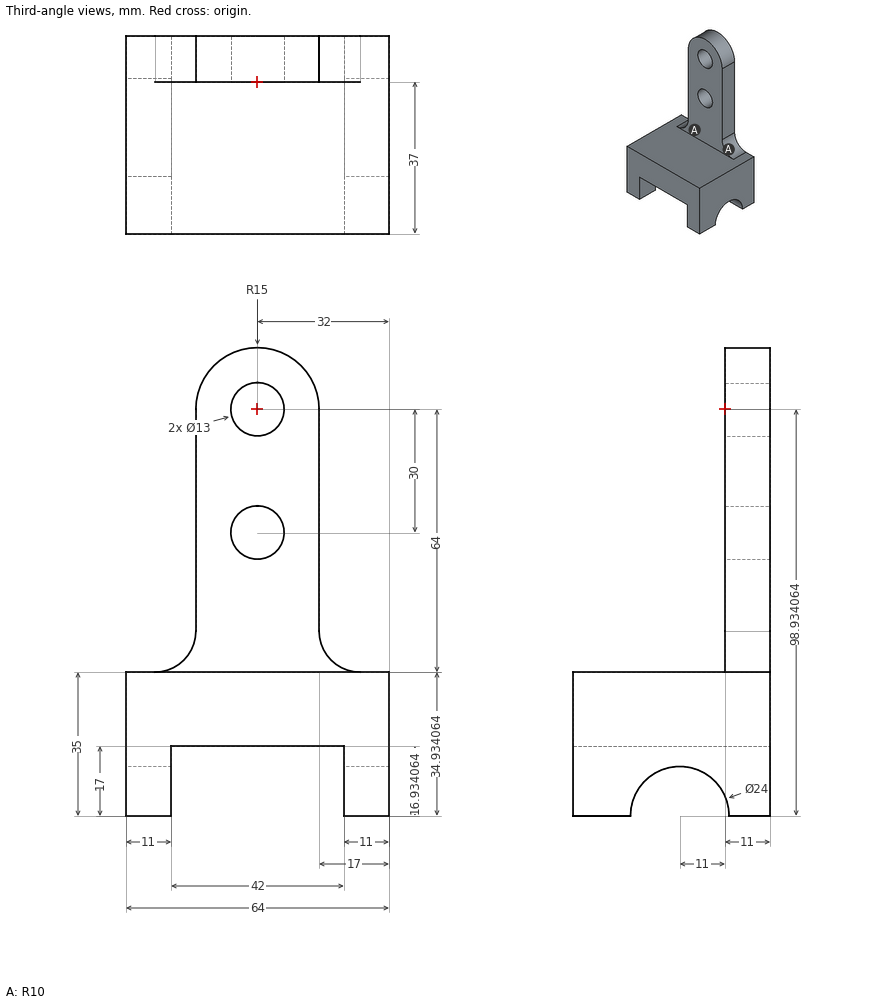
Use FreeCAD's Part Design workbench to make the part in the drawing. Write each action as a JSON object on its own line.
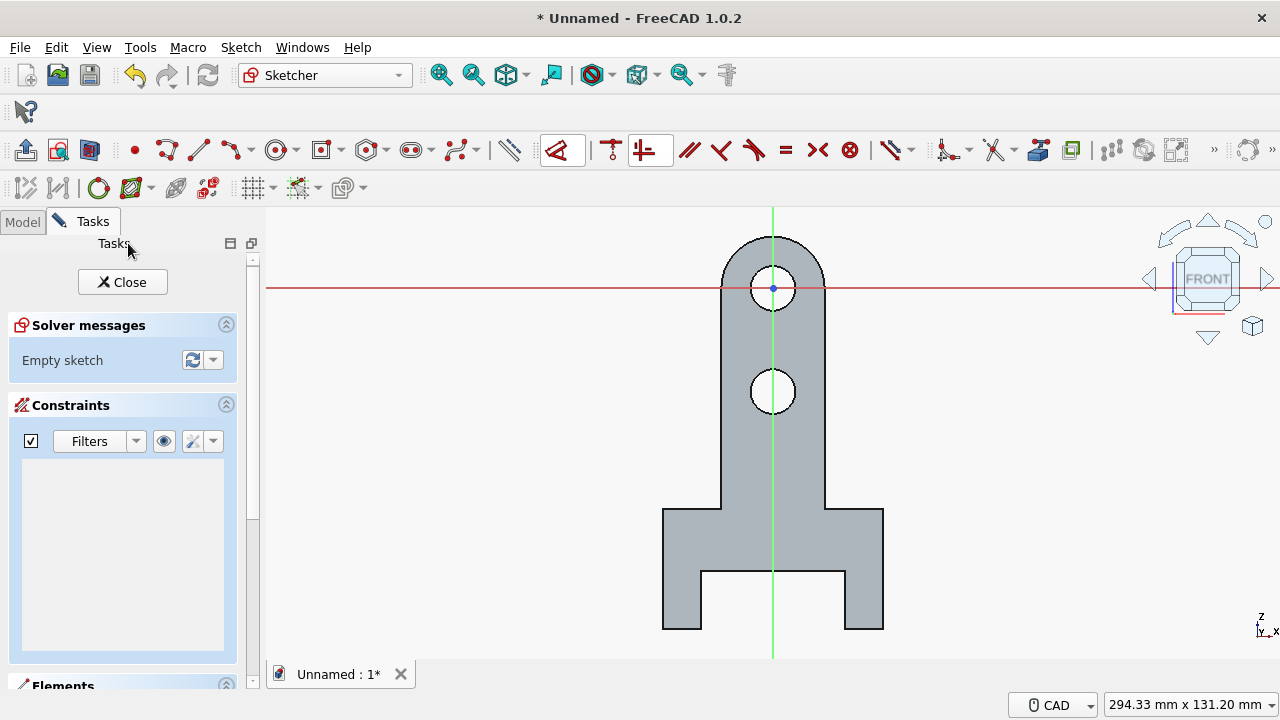
{"action": "scroll", "coordinate": [395, 316], "scroll_direction": "down", "scroll_amount": 1}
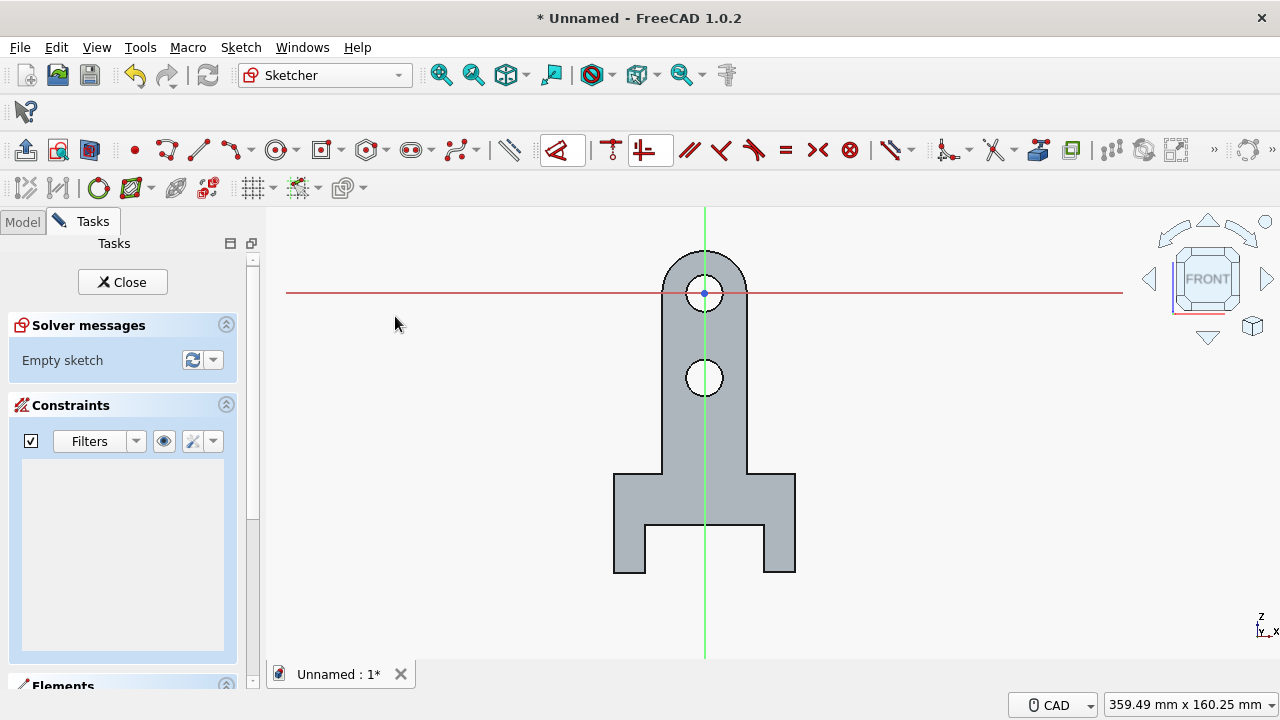
{"action": "left_click", "coordinate": [168, 150]}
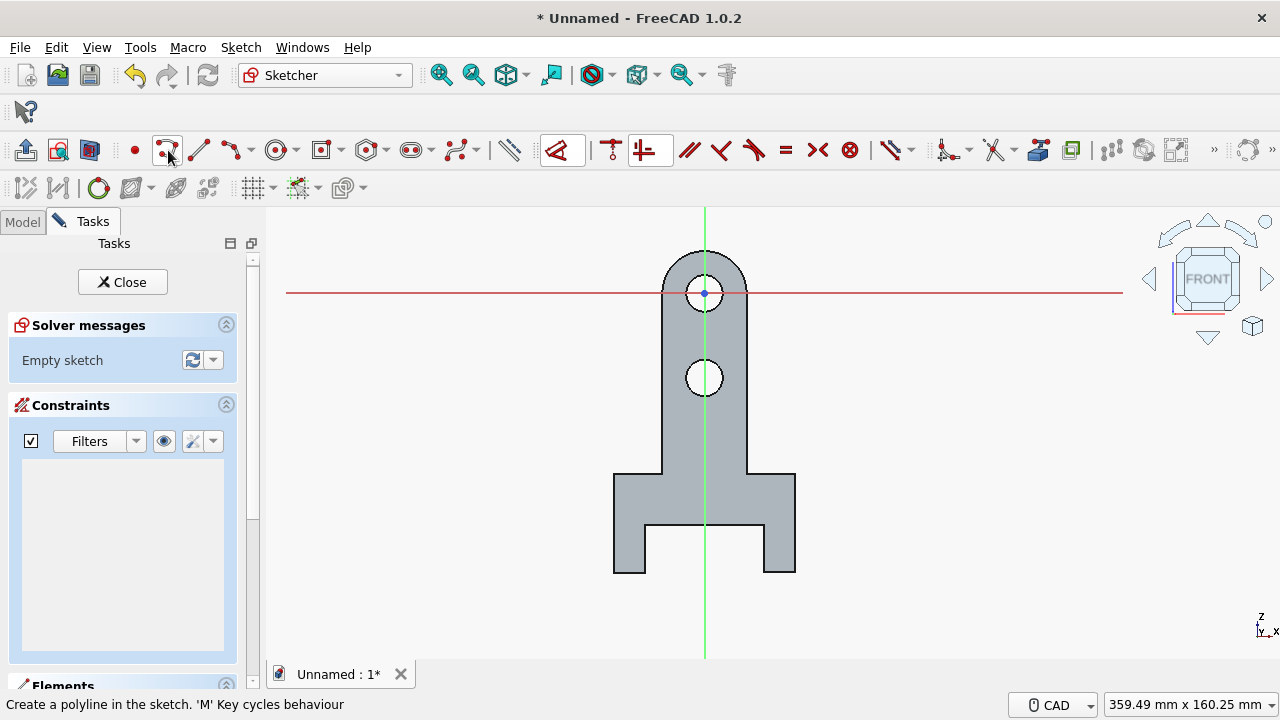
{"action": "left_click", "coordinate": [795, 474]}
{"action": "left_click", "coordinate": [614, 474]}
{"action": "left_click", "coordinate": [614, 573]}
{"action": "left_click", "coordinate": [645, 573]}
{"action": "left_click", "coordinate": [645, 525]}
{"action": "left_click", "coordinate": [764, 525]}
{"action": "left_click", "coordinate": [764, 572]}
{"action": "left_click", "coordinate": [795, 572]}
{"action": "left_click", "coordinate": [795, 475]}
{"action": "key", "text": "Escape"}
{"action": "key", "text": "Escape"}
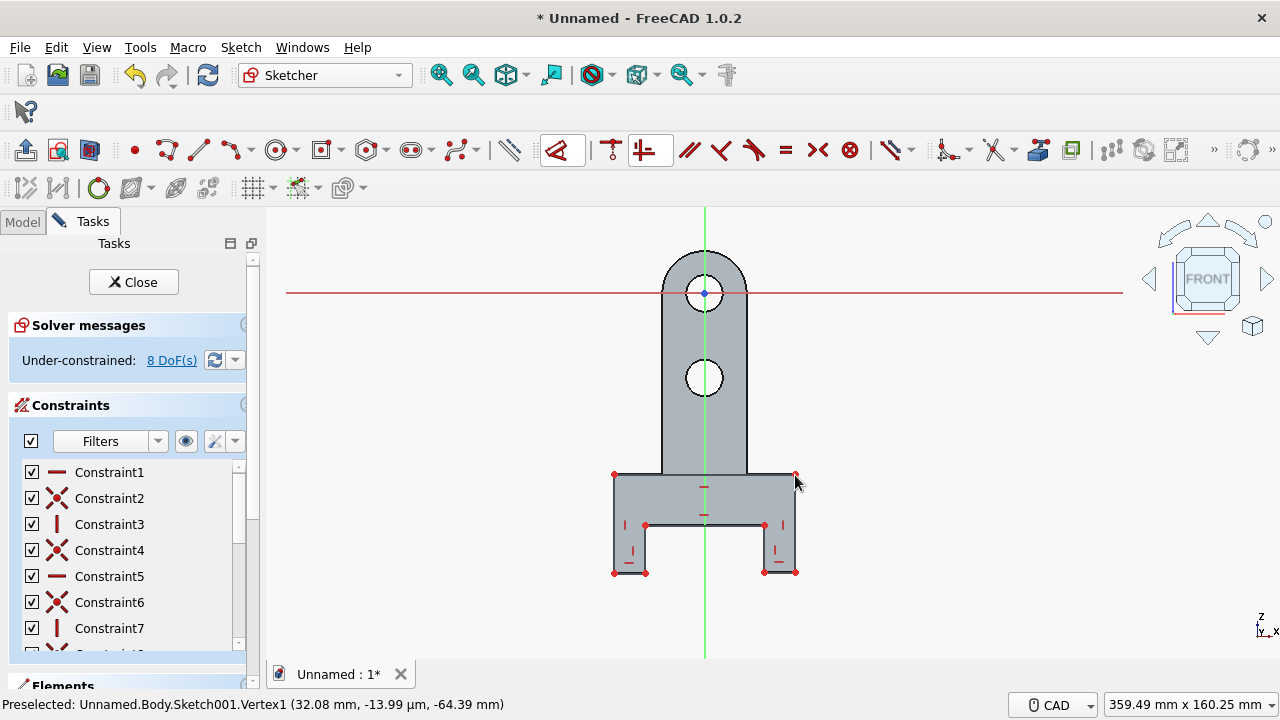
{"action": "left_click", "coordinate": [741, 475]}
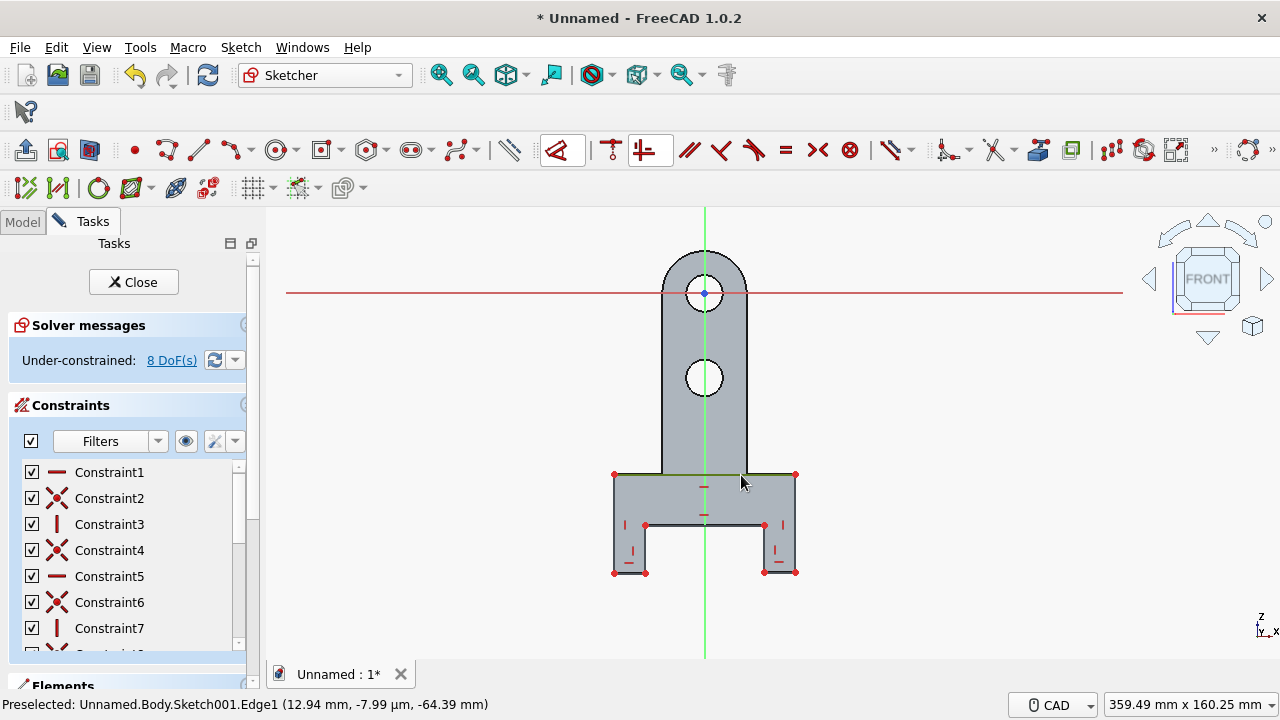
{"action": "key", "text": "l"}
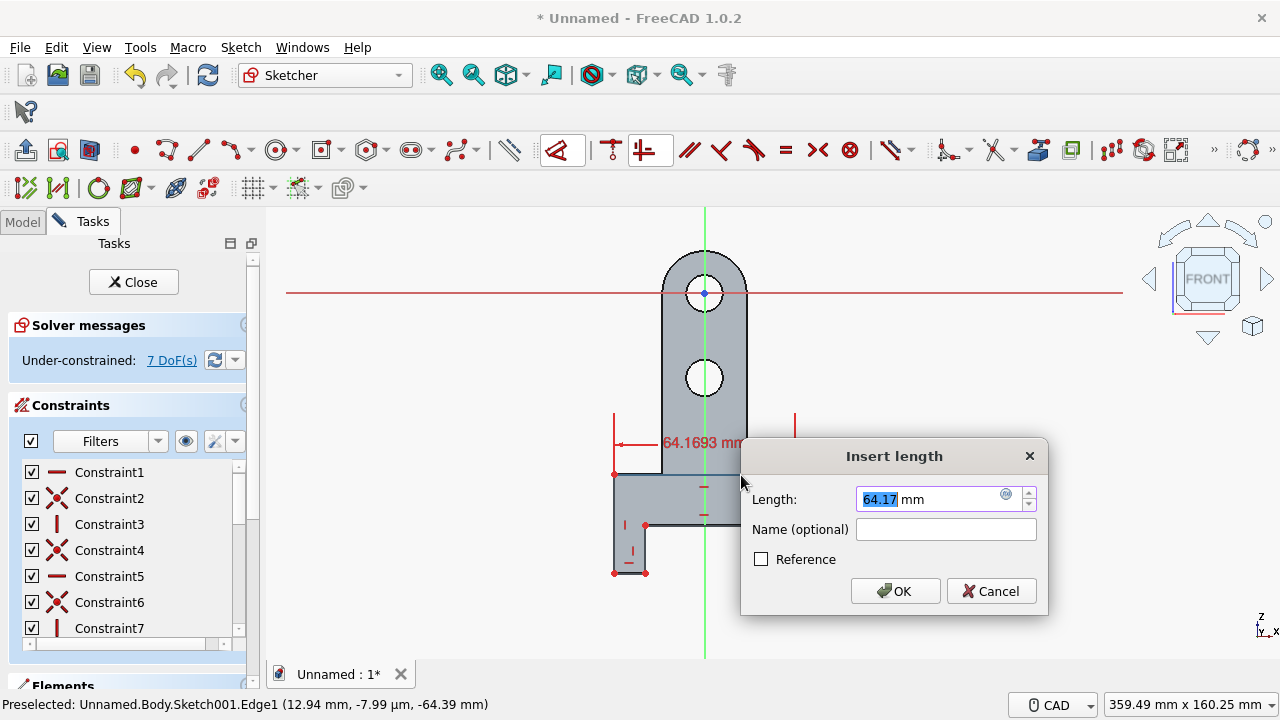
{"action": "type", "text": "64"}
{"action": "key", "text": "Return"}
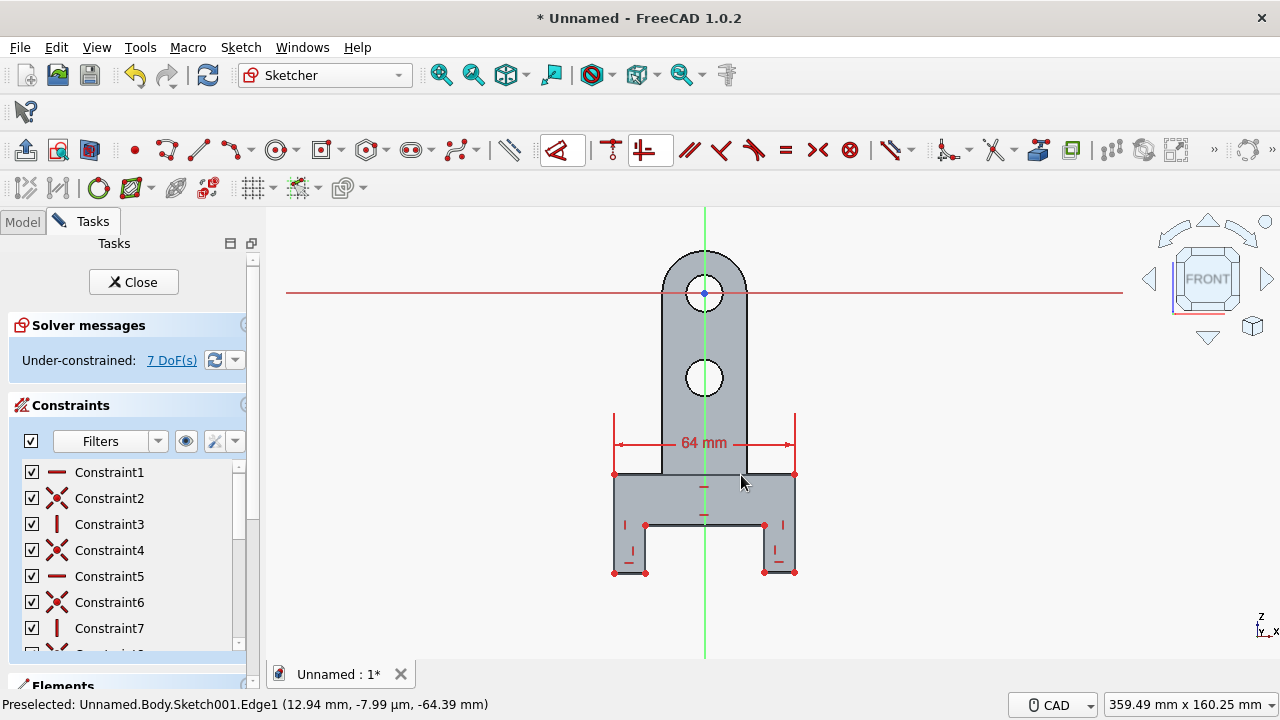
{"action": "left_click", "coordinate": [614, 505]}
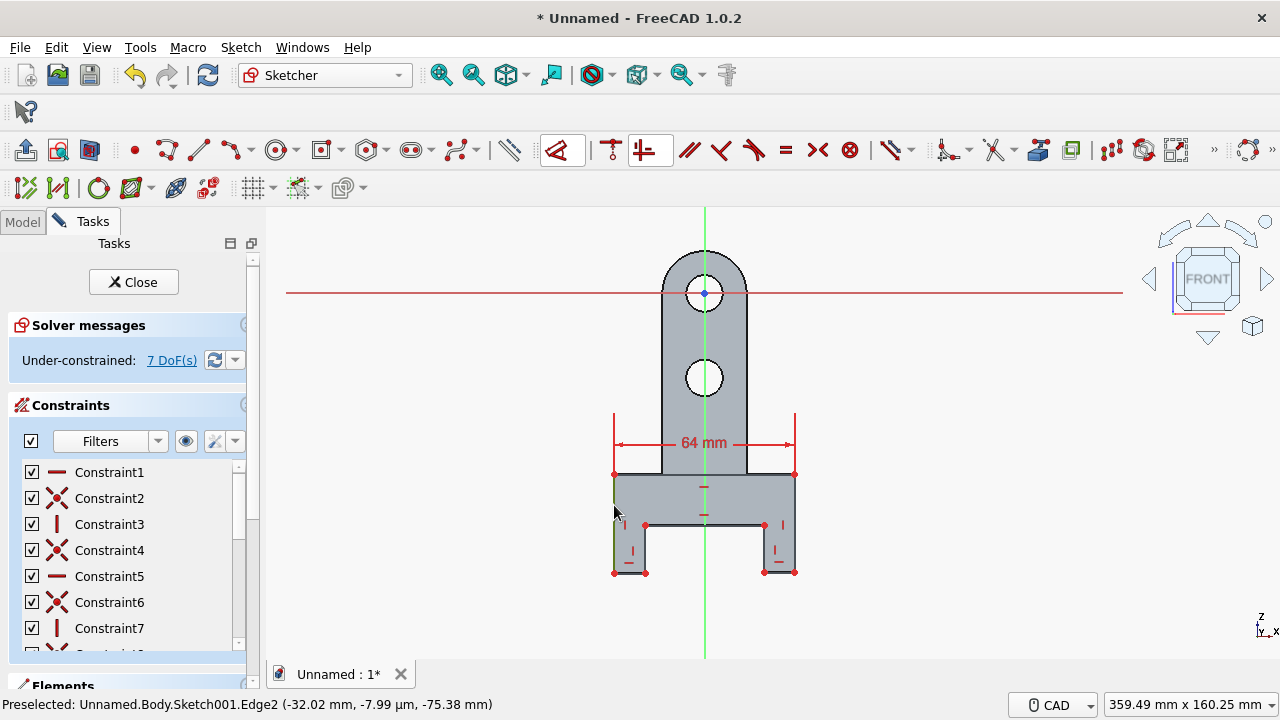
{"action": "left_click", "coordinate": [580, 150]}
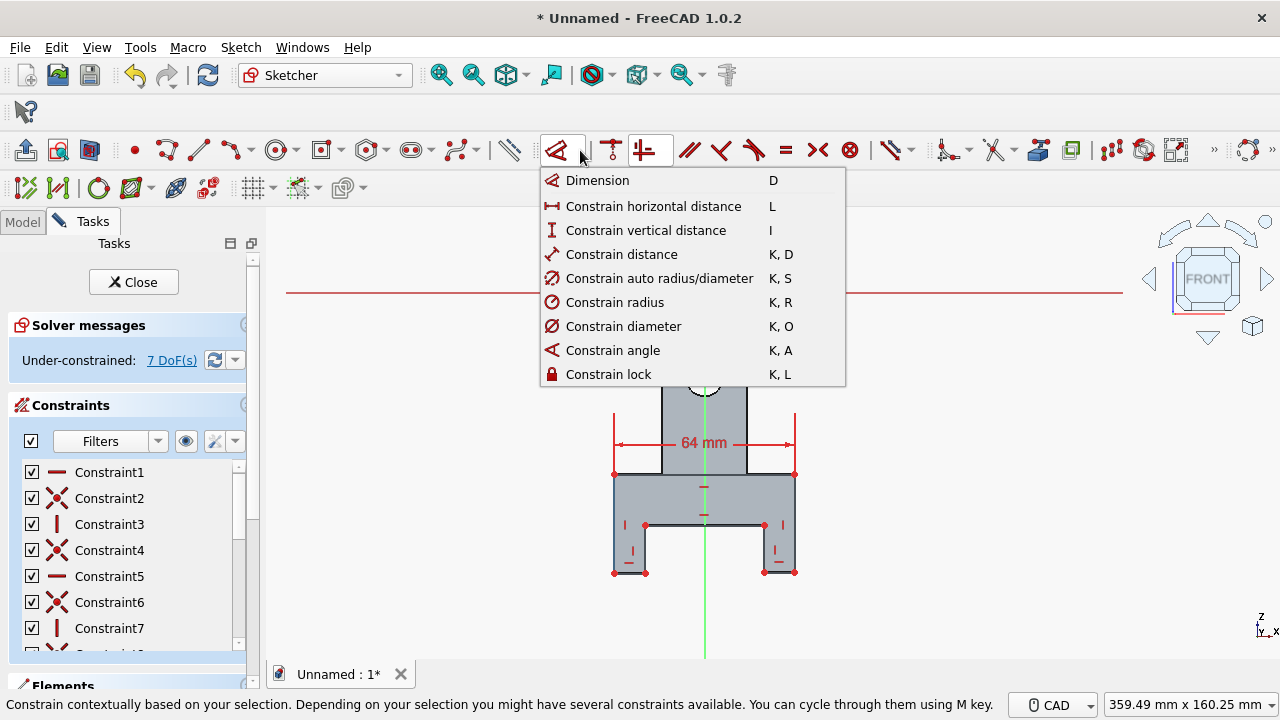
{"action": "left_click", "coordinate": [693, 230]}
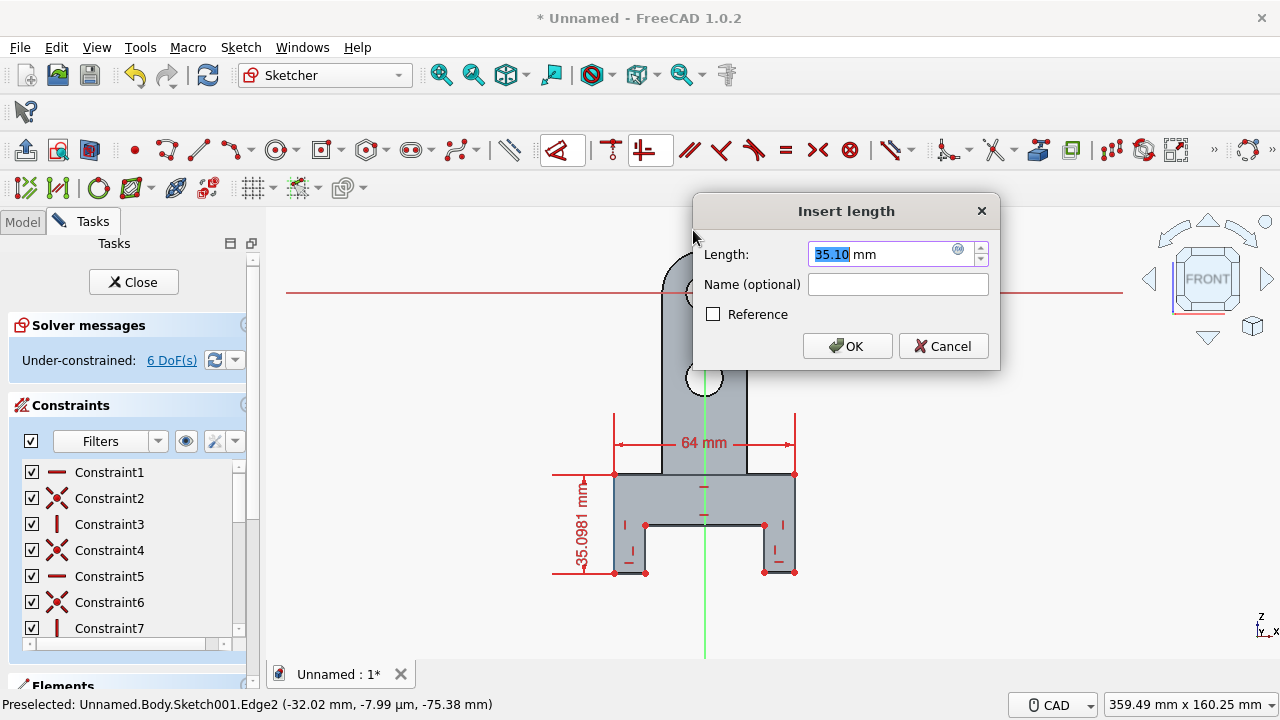
{"action": "type", "text": "35"}
{"action": "key", "text": "Return"}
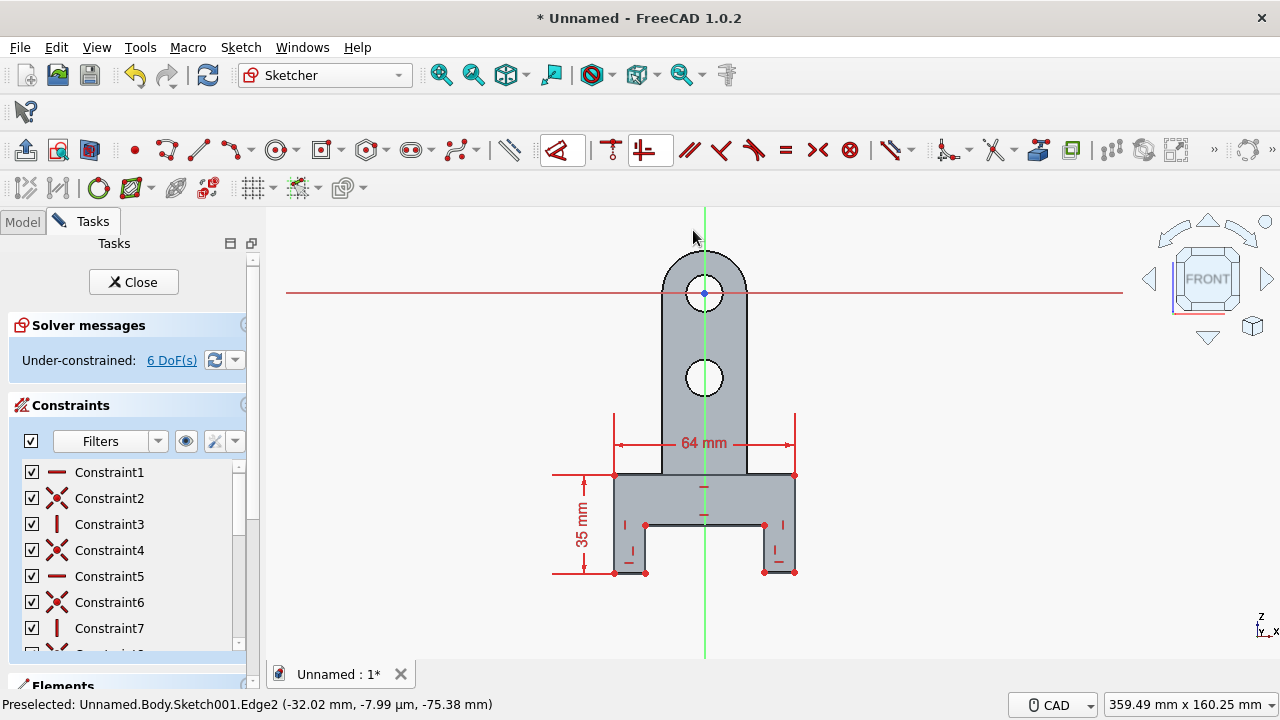
{"action": "scroll", "coordinate": [623, 574], "scroll_direction": "up", "scroll_amount": 3}